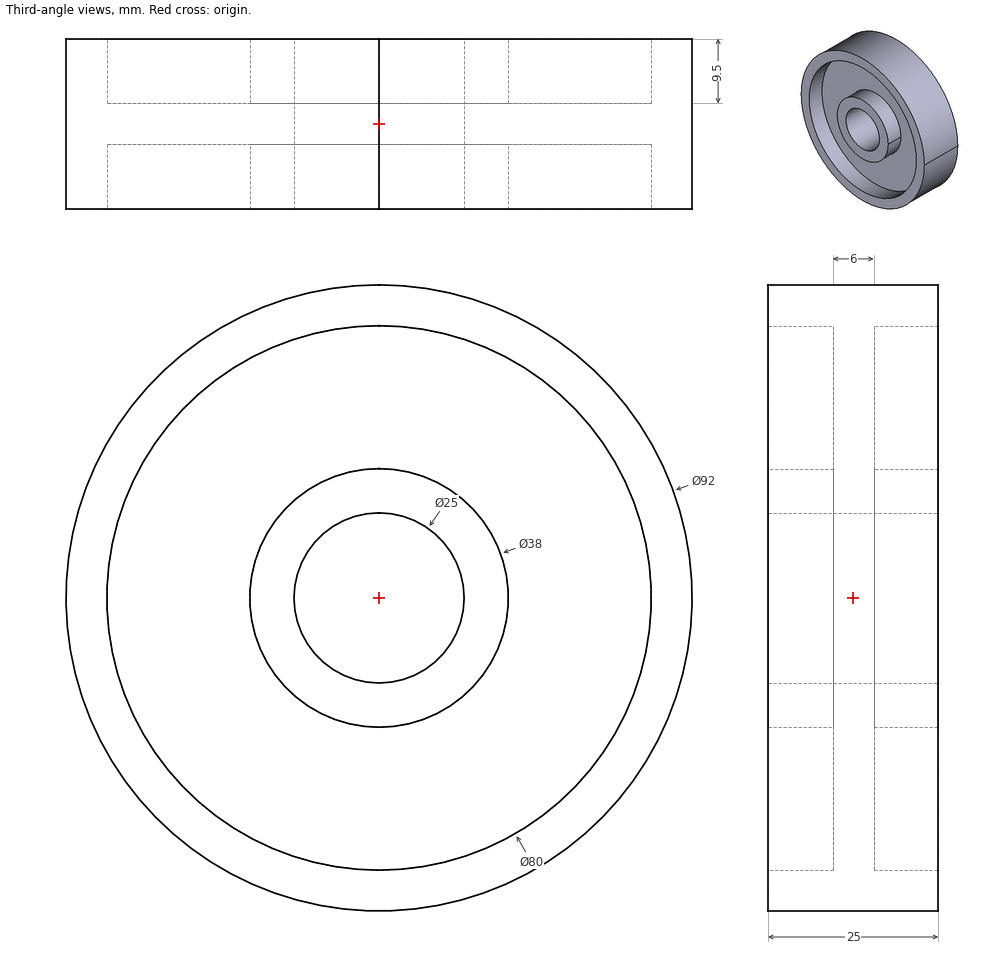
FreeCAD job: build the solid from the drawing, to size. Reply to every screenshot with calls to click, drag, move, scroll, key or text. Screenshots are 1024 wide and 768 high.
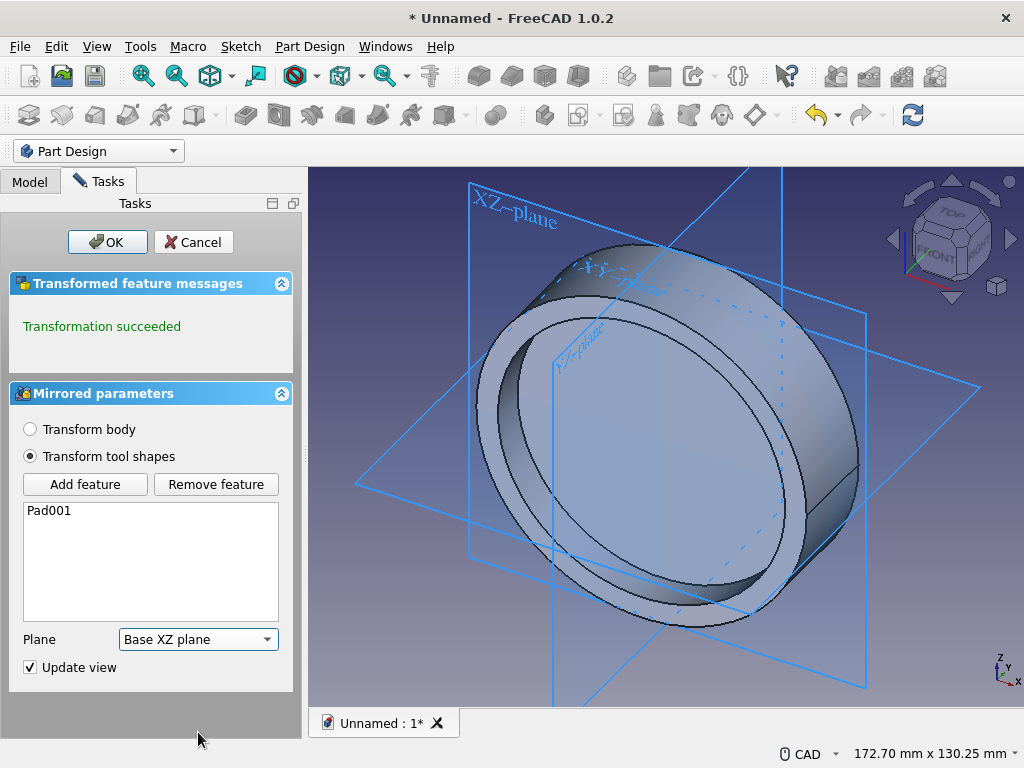
click(108, 242)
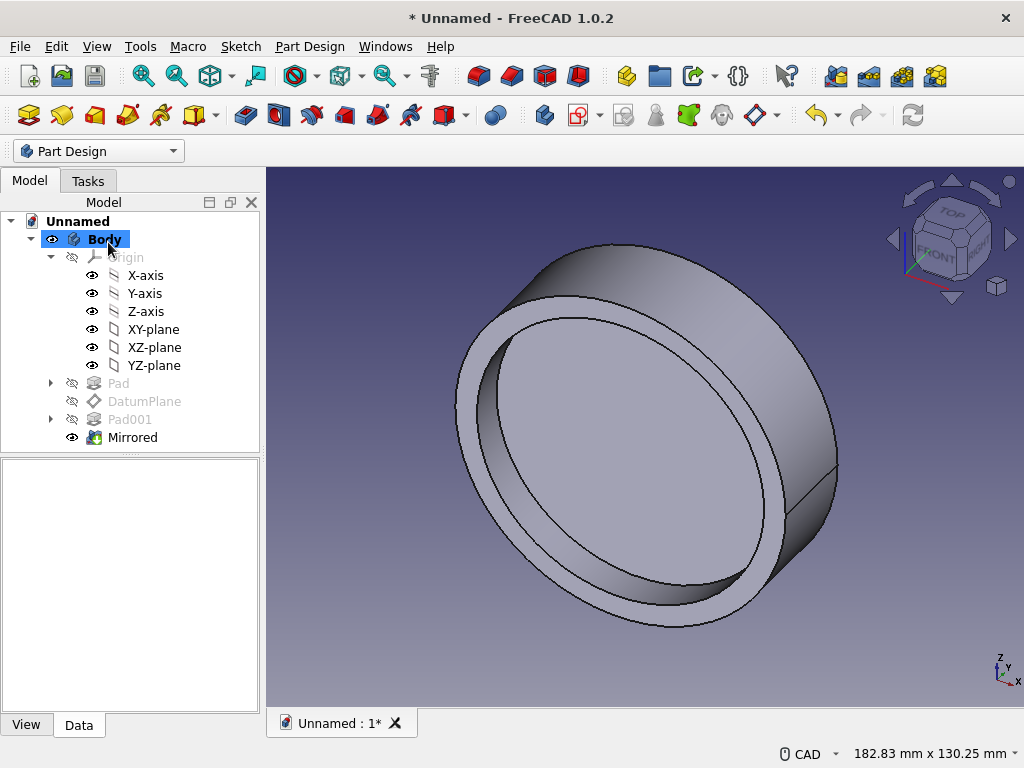
key(4)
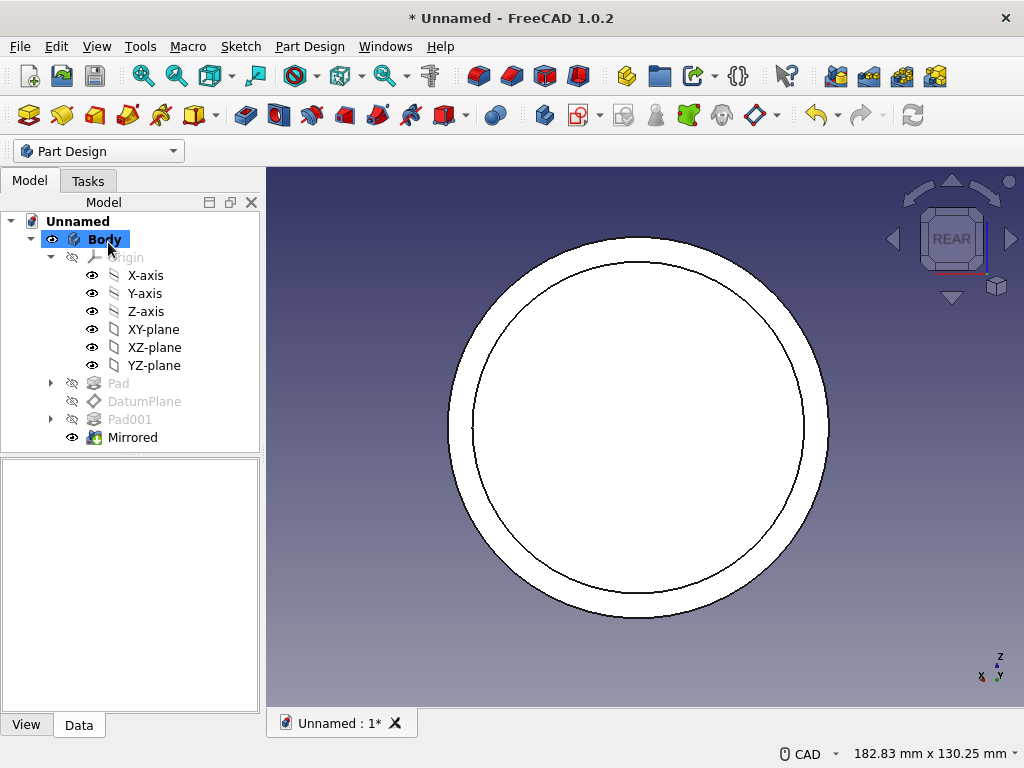
click(584, 590)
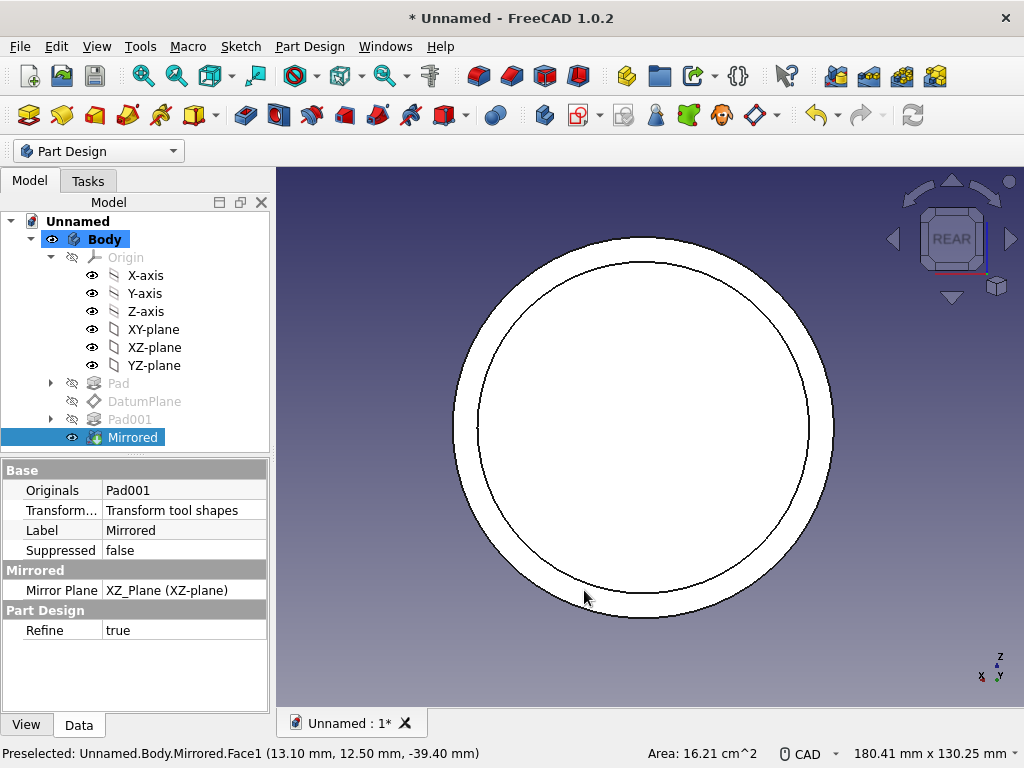
click(578, 116)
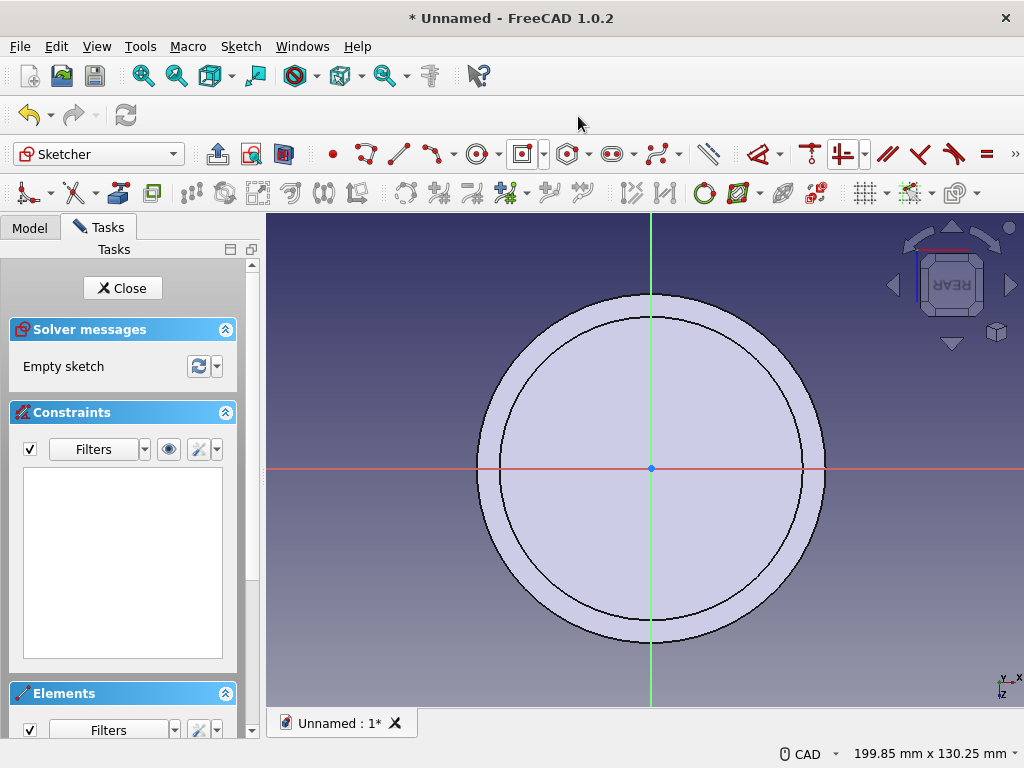
scroll(712, 476, up, 4)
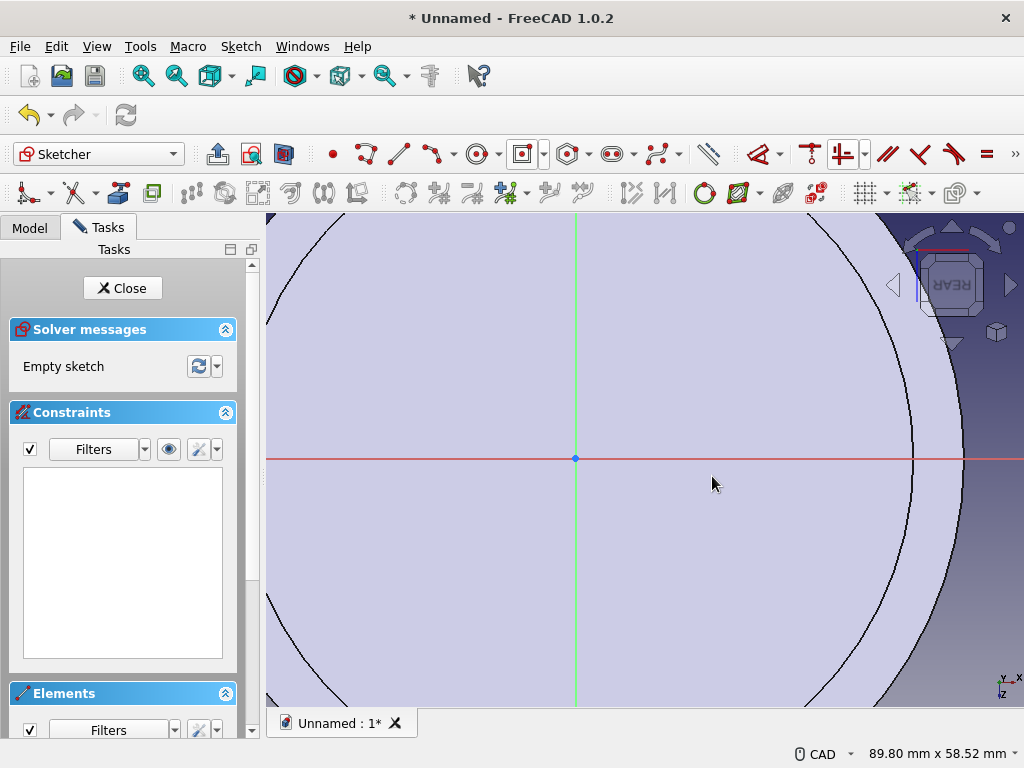
click(476, 154)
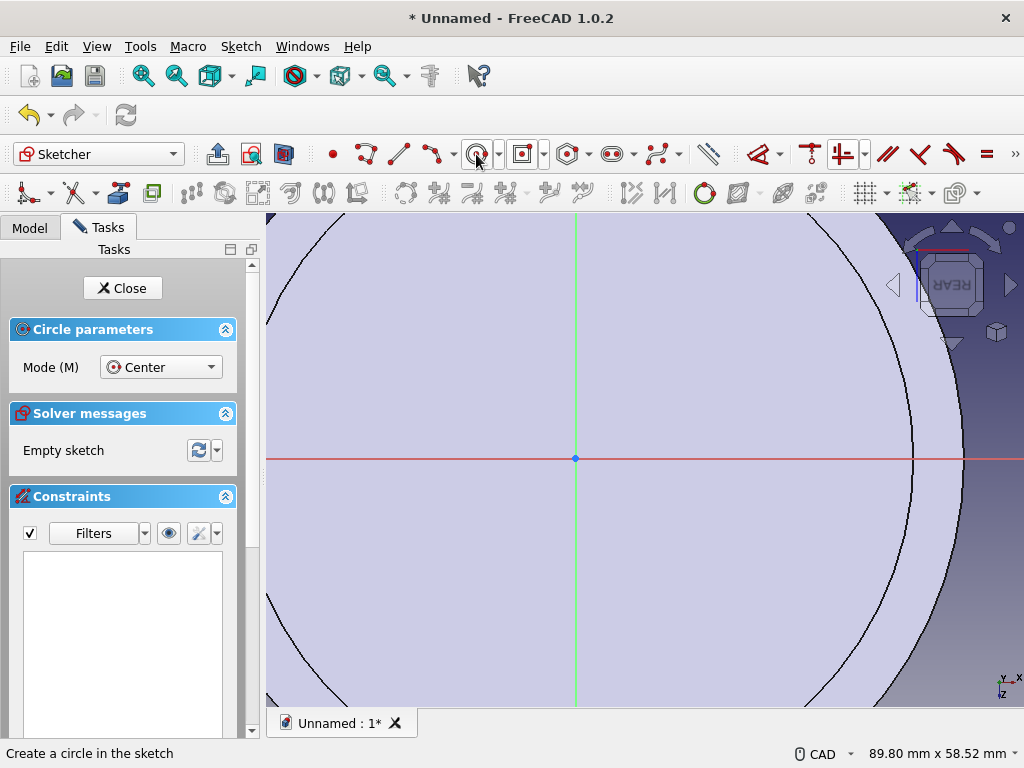
click(576, 459)
move(689, 345)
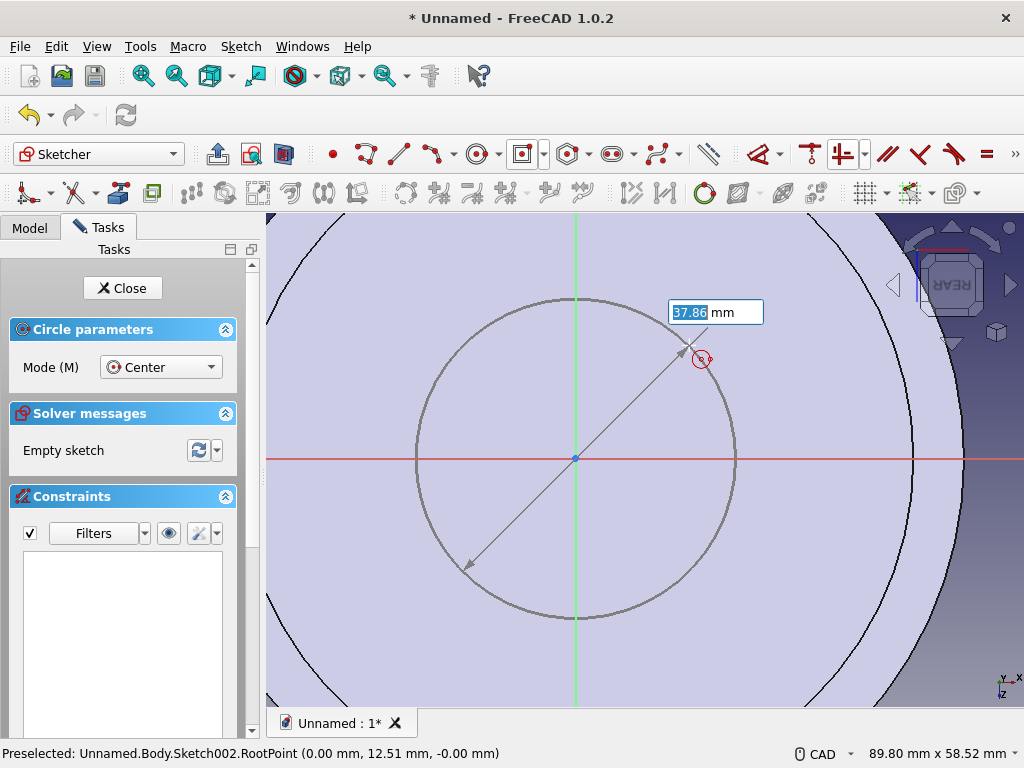
text(38)
key(Return)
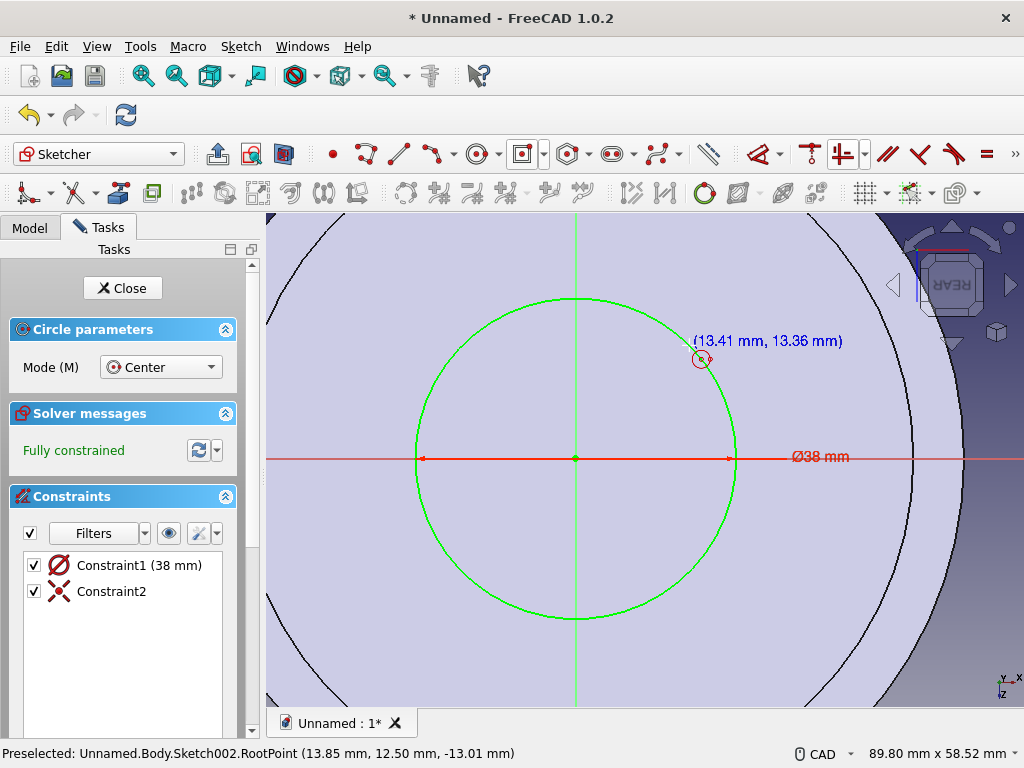
click(576, 459)
move(650, 384)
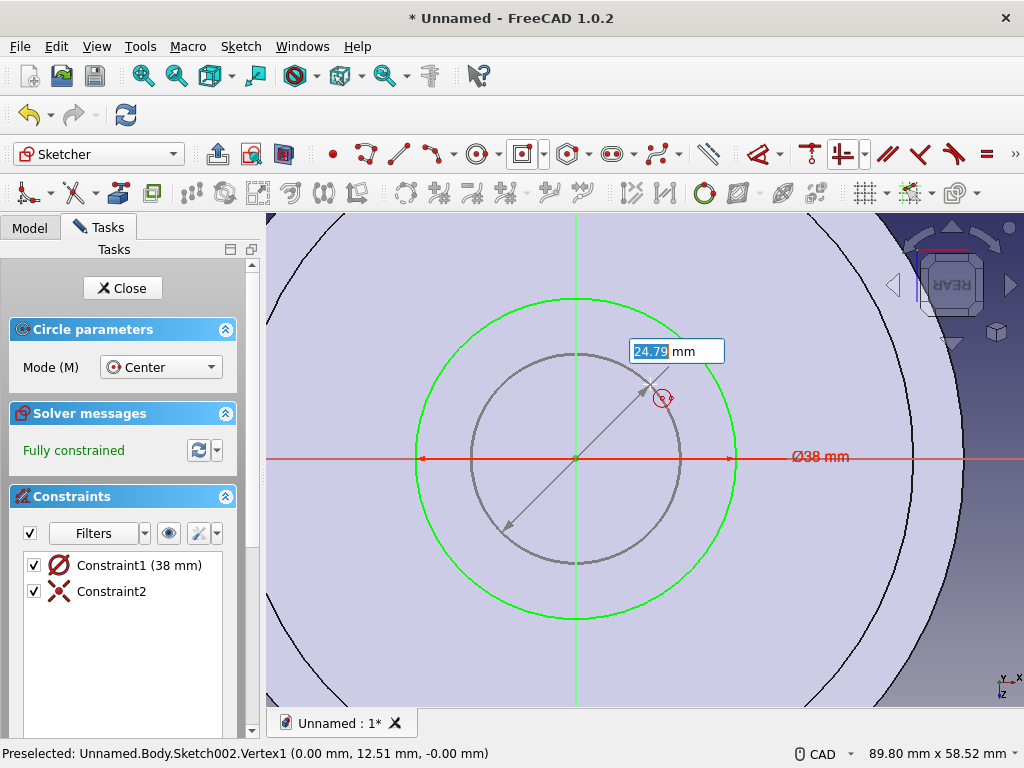
text(25)
key(Return)
key(Escape)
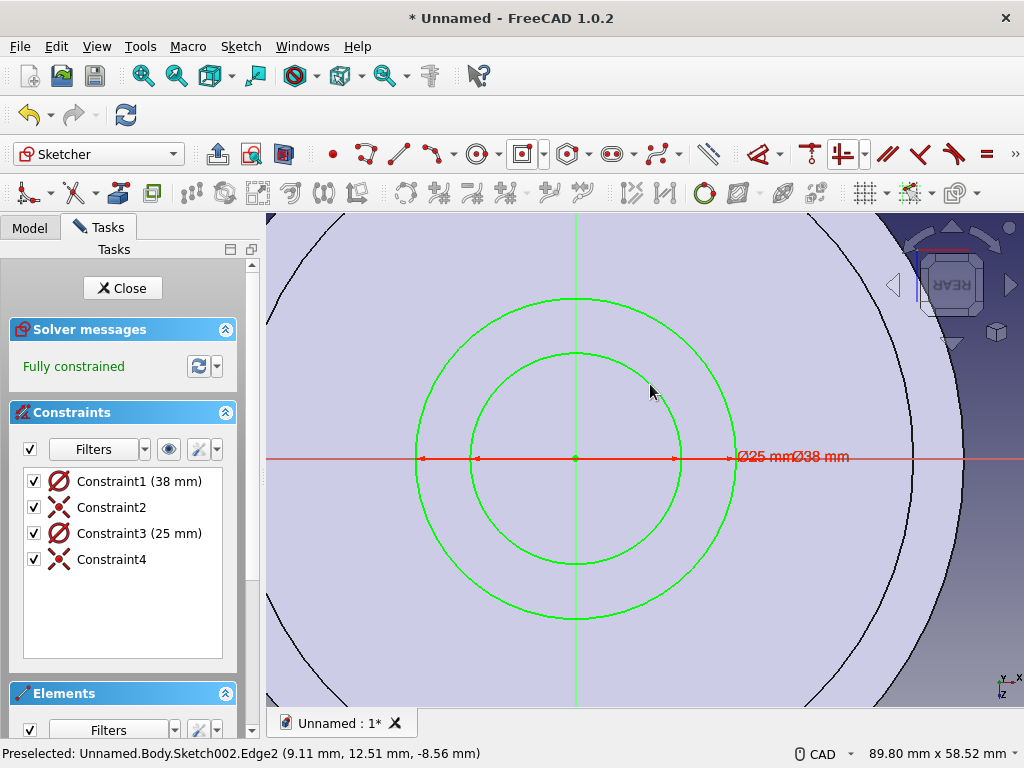
click(123, 288)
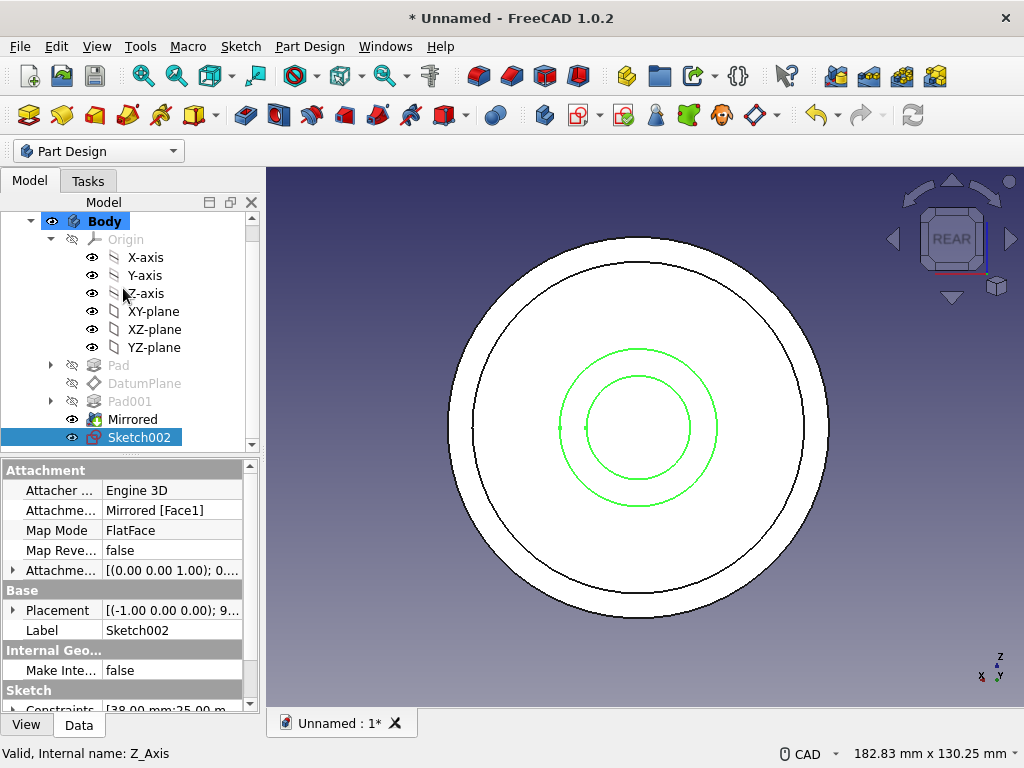
click(29, 116)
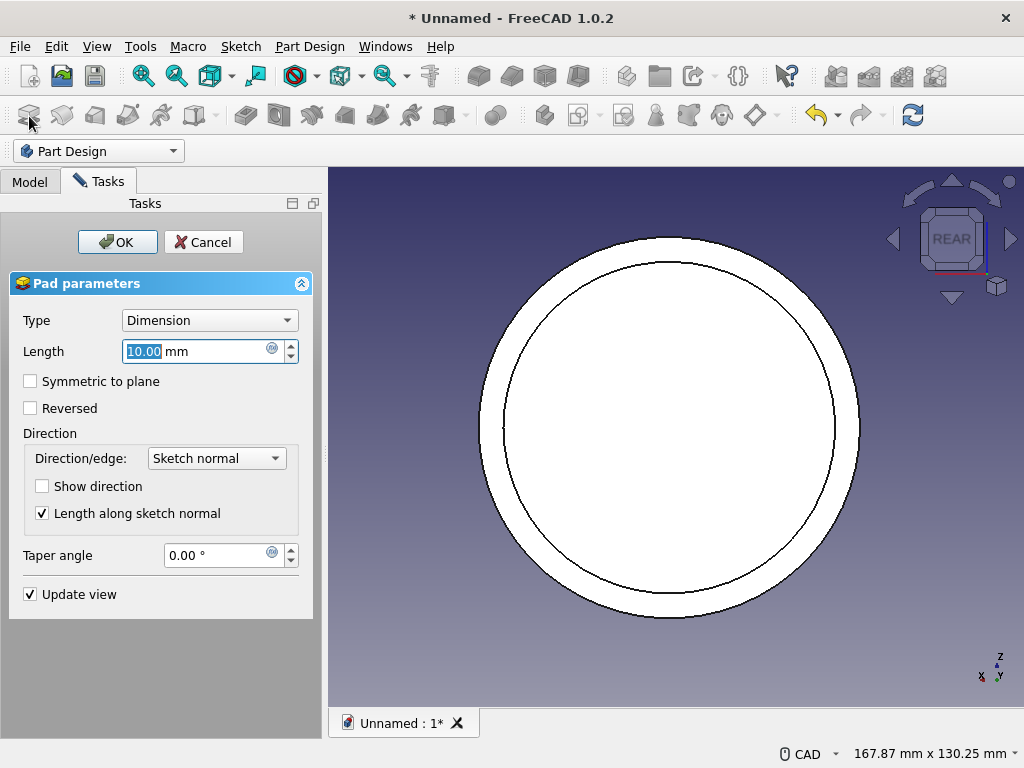
text(25)
key(Tab)